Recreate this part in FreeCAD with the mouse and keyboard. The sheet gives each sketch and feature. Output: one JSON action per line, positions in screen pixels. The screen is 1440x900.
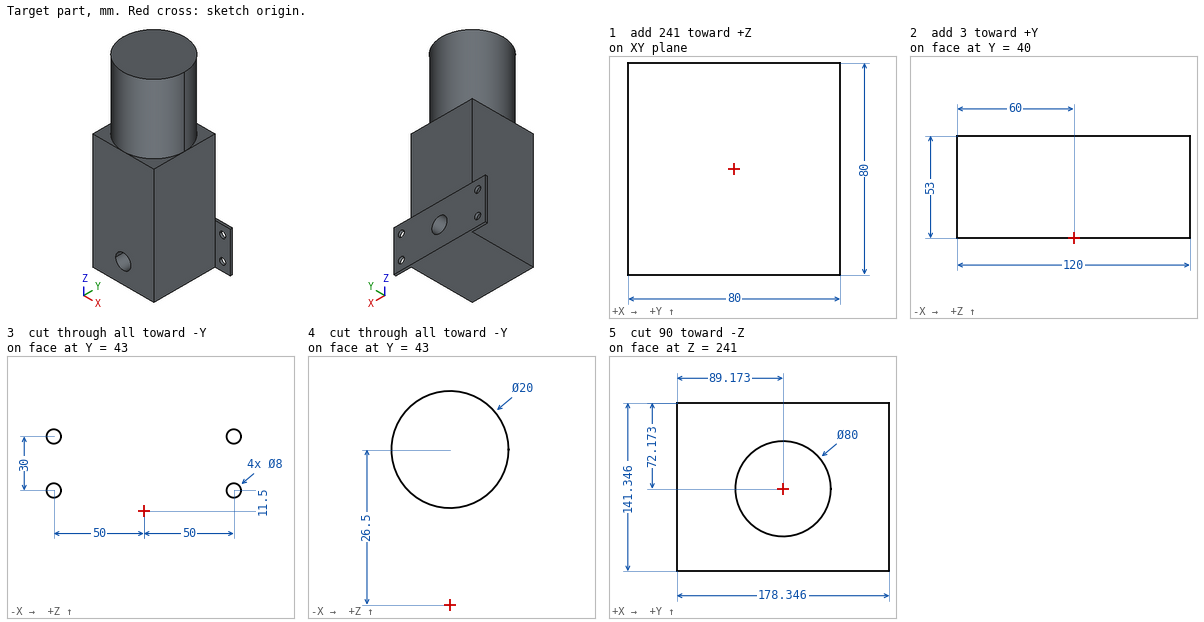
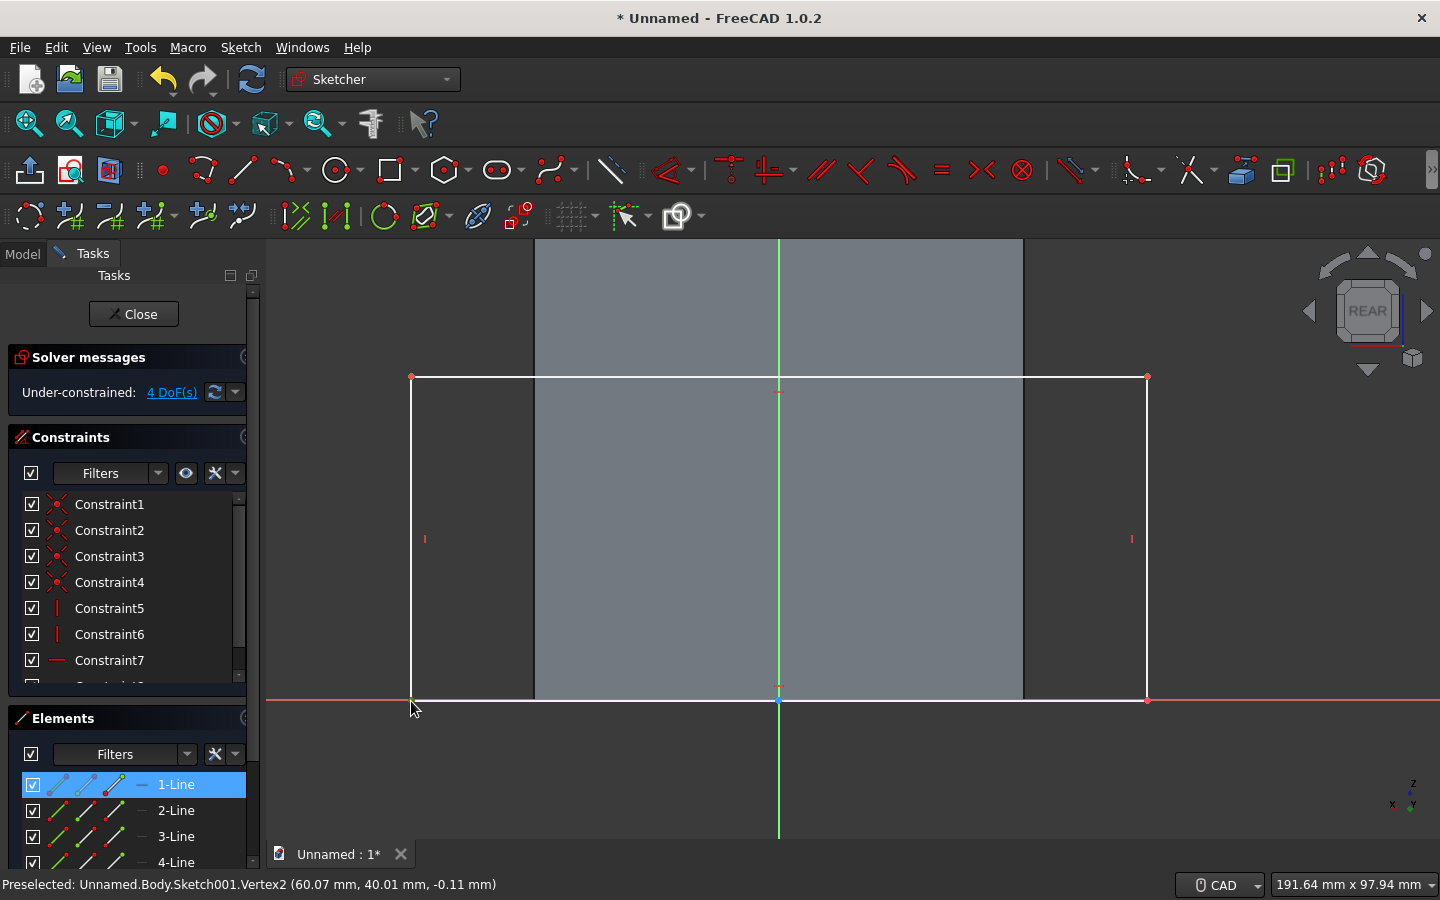
{"action": "left_click", "coordinate": [364, 700]}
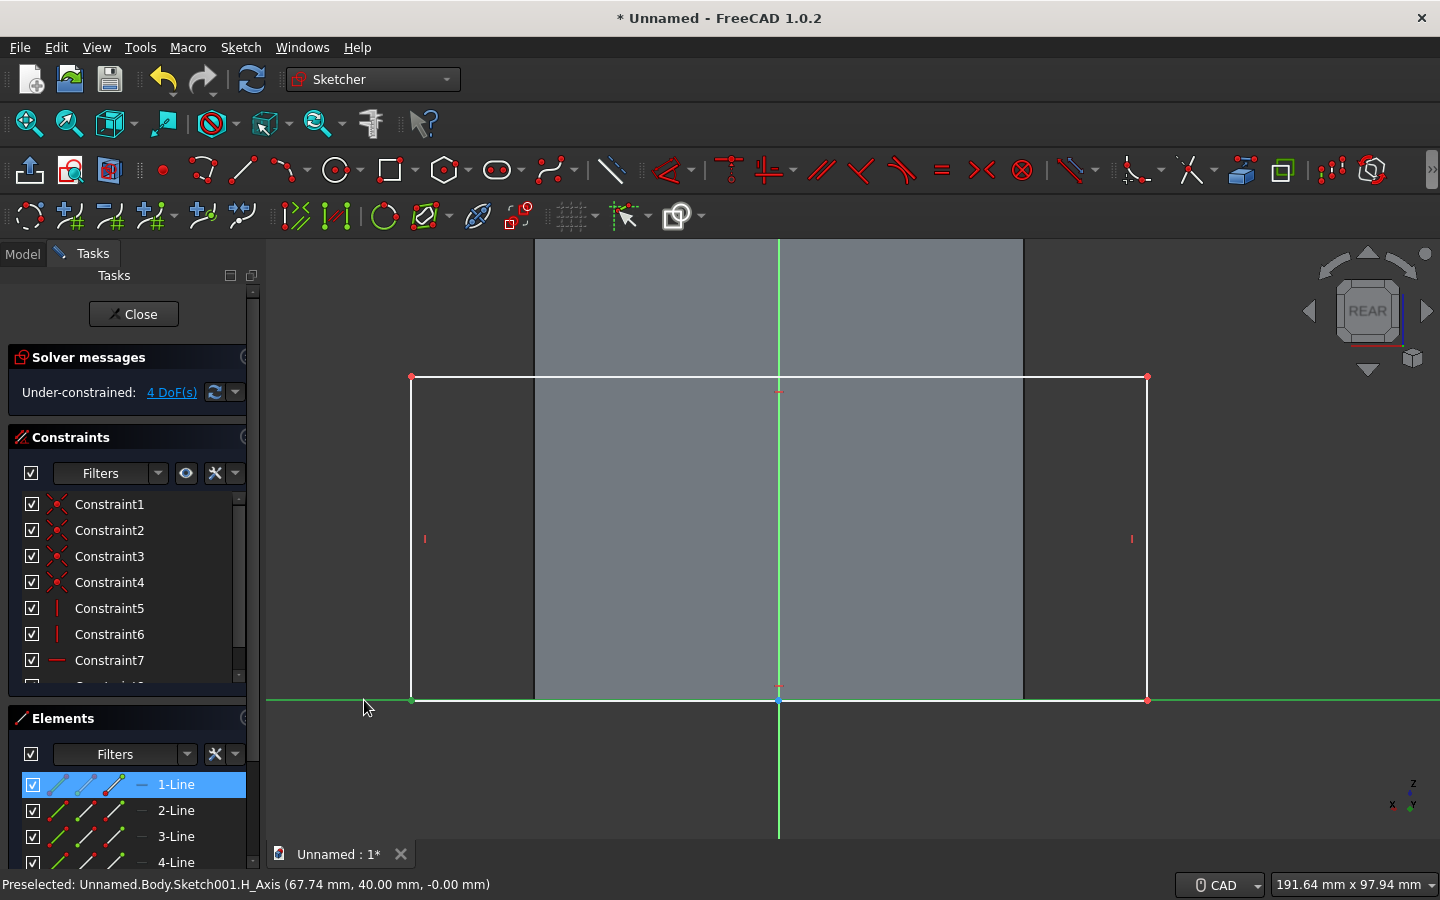
{"action": "key", "text": "c"}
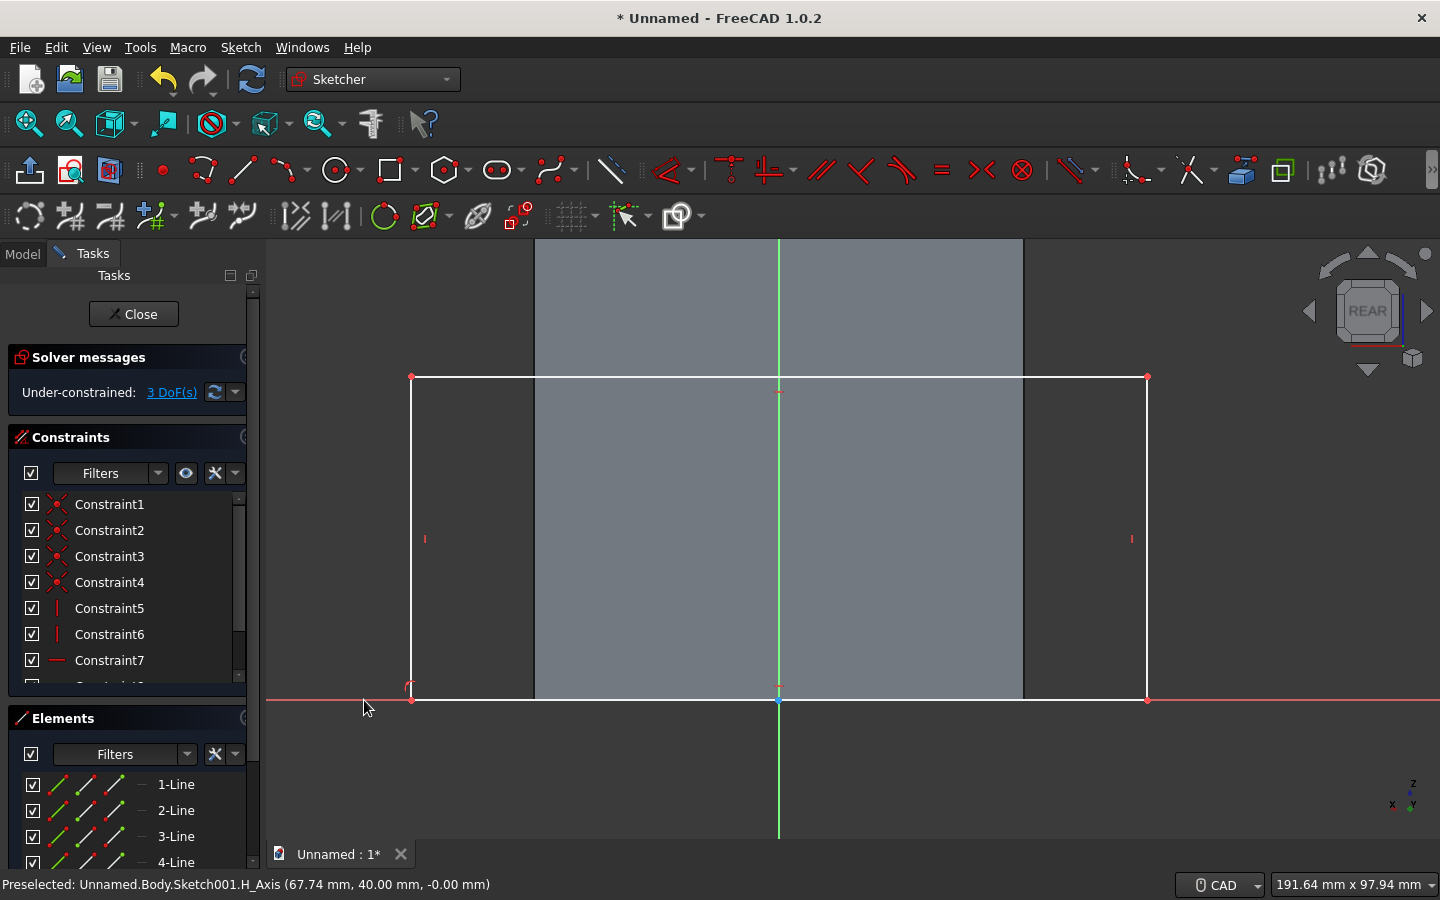
{"action": "left_click", "coordinate": [666, 170]}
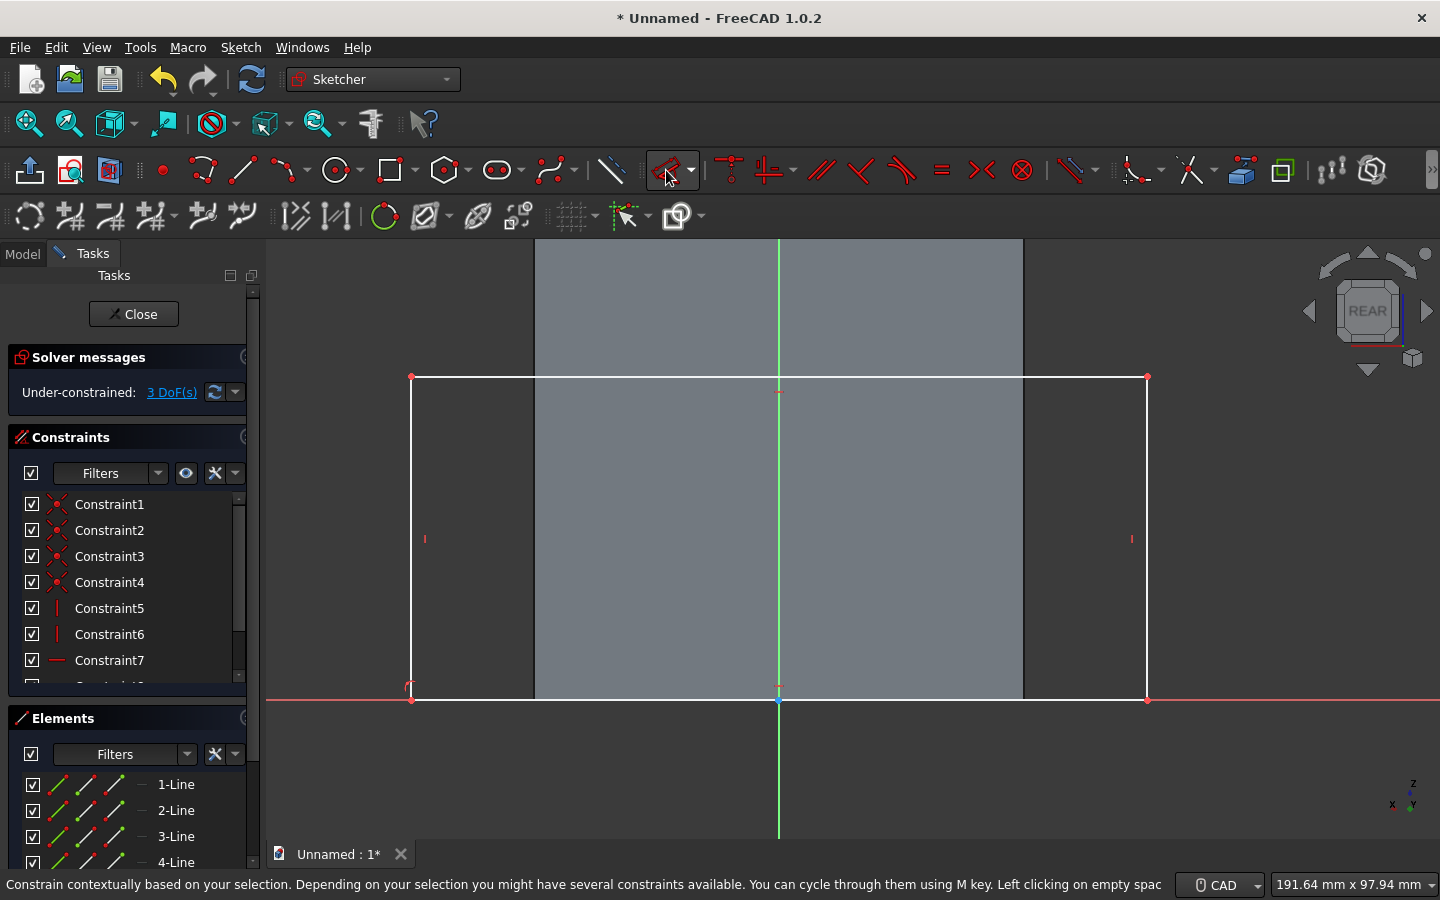
{"action": "left_click", "coordinate": [411, 474]}
{"action": "left_click", "coordinate": [377, 539]}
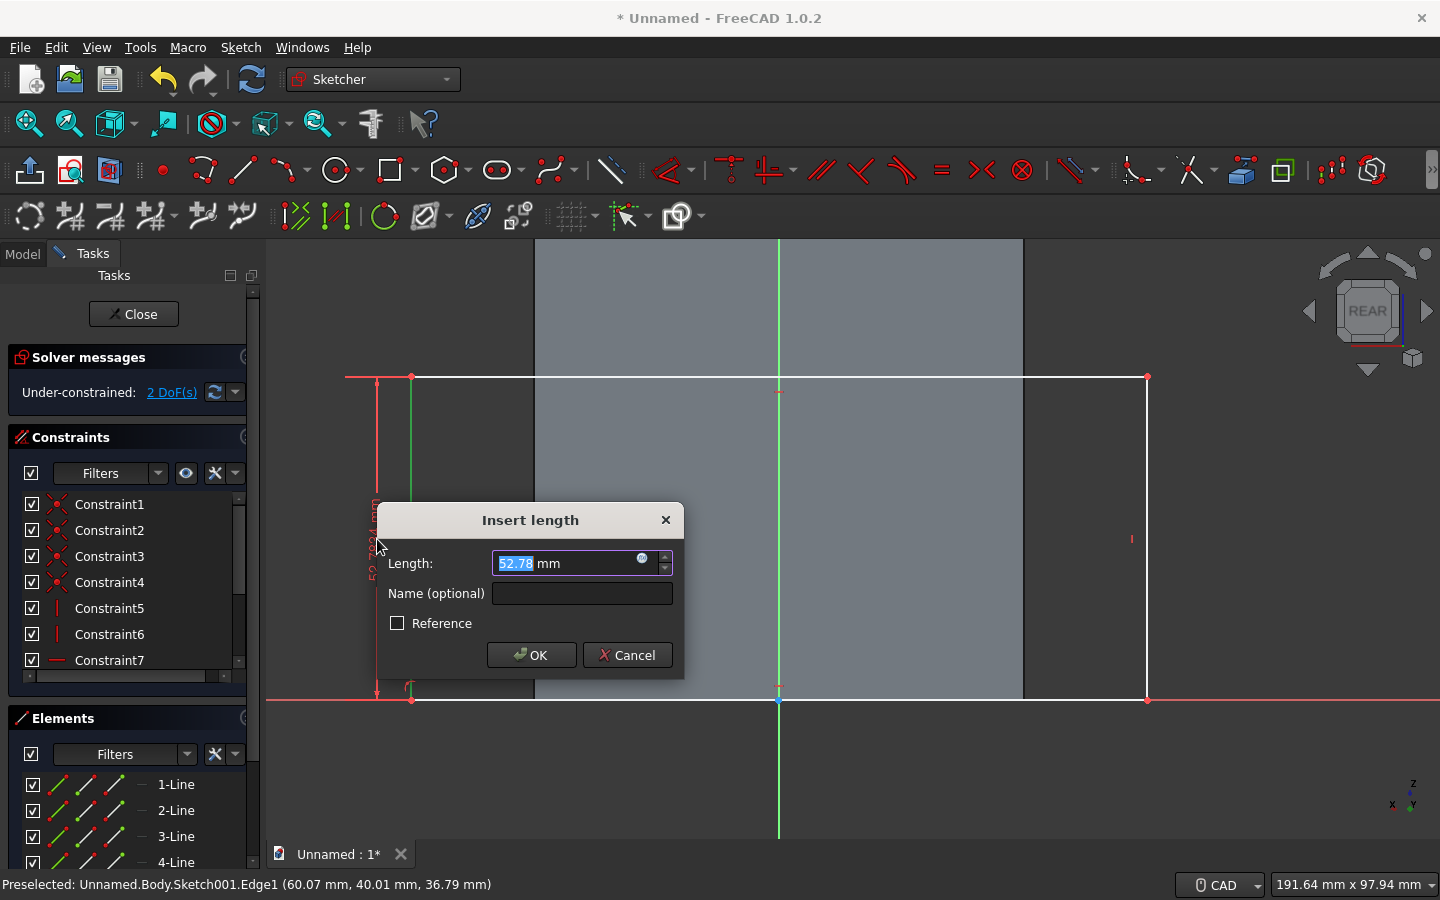
{"action": "type", "text": "53"}
{"action": "key", "text": "Return"}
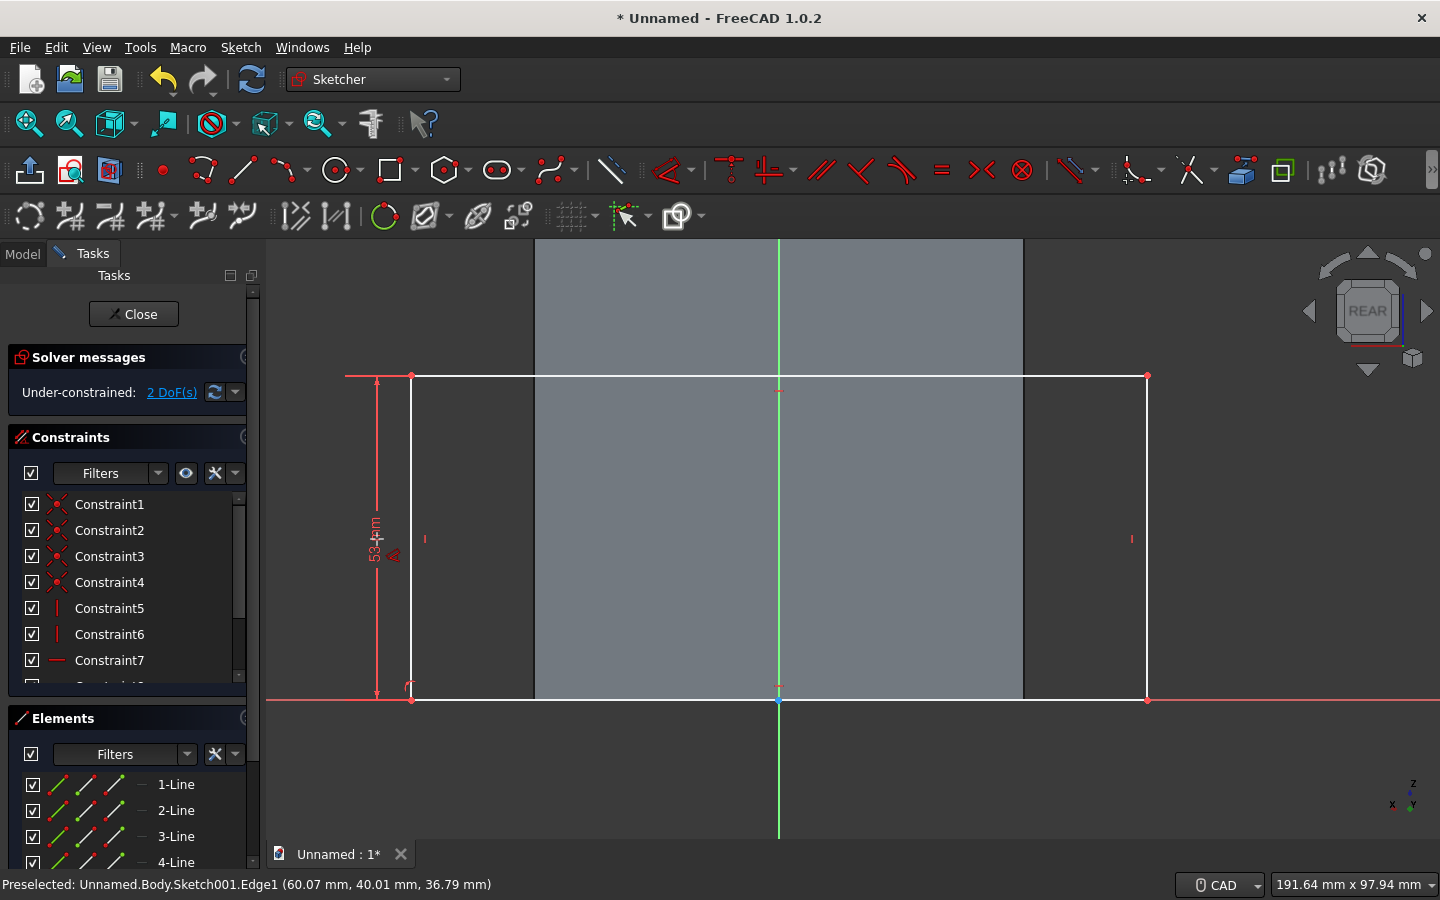
{"action": "left_click", "coordinate": [632, 700]}
{"action": "left_click", "coordinate": [610, 734]}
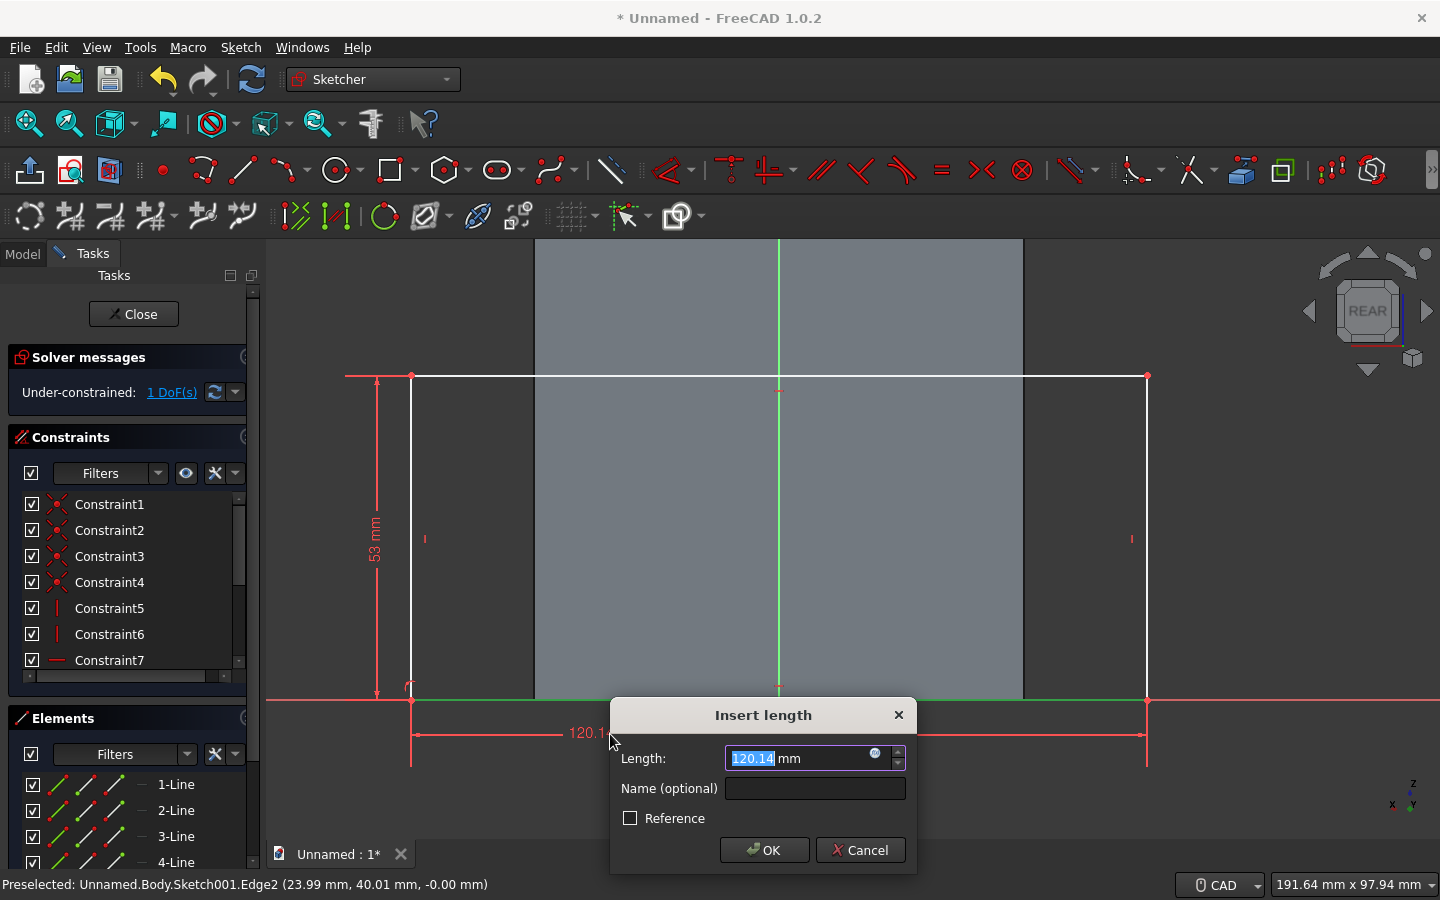
{"action": "type", "text": "120"}
{"action": "key", "text": "Return"}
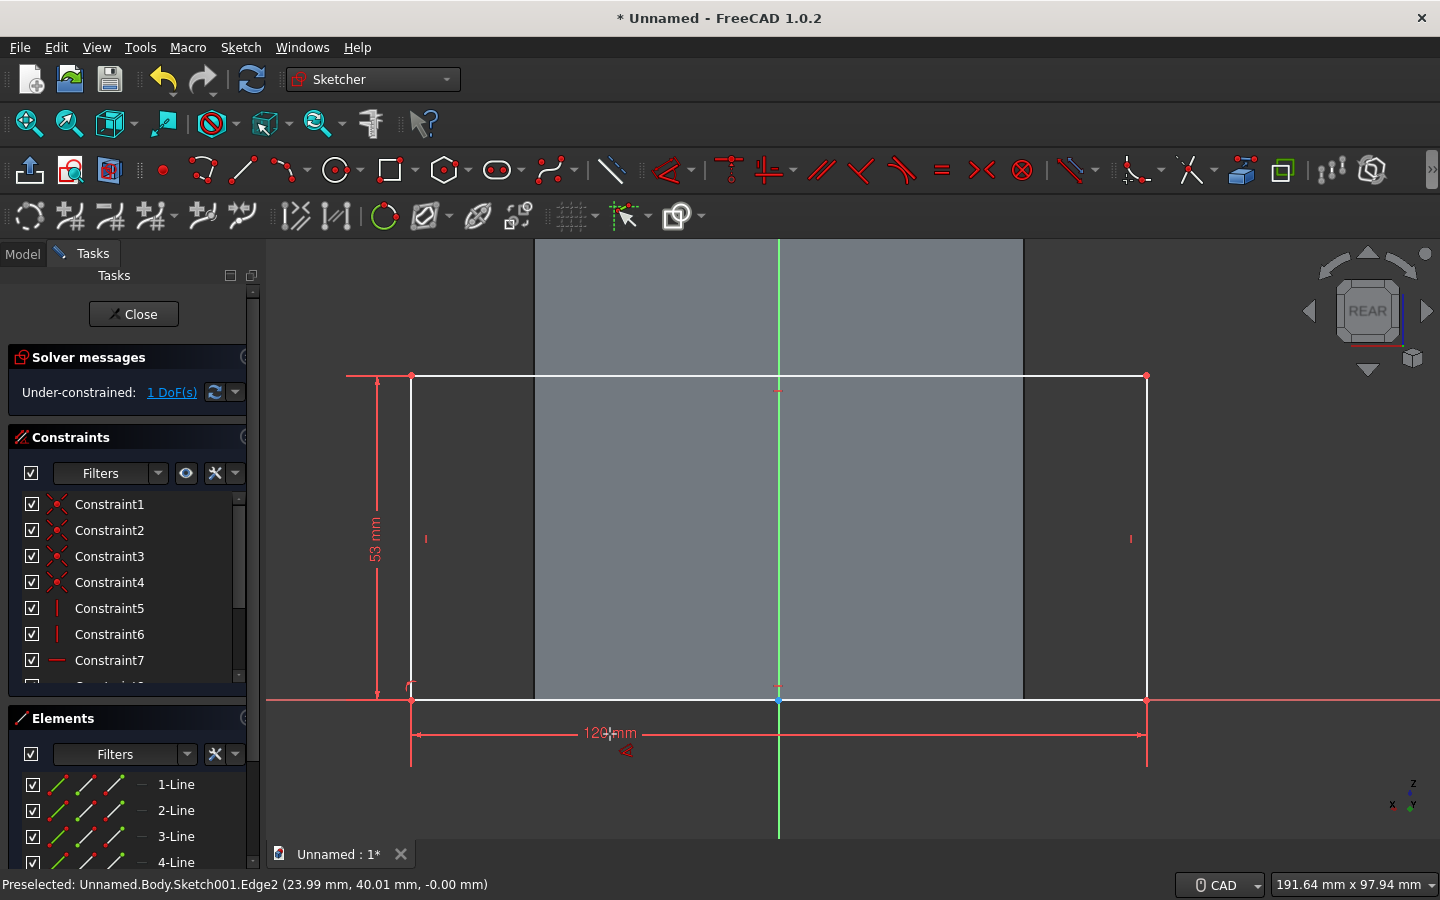
{"action": "left_click", "coordinate": [411, 376]}
{"action": "left_click", "coordinate": [511, 734]}